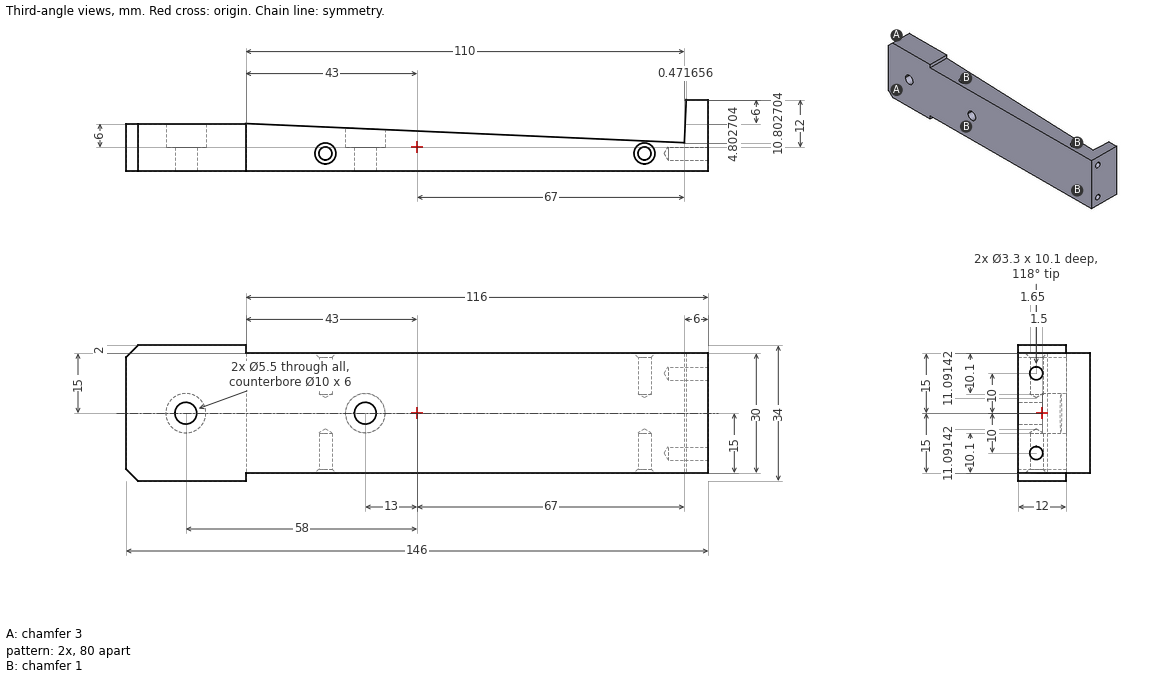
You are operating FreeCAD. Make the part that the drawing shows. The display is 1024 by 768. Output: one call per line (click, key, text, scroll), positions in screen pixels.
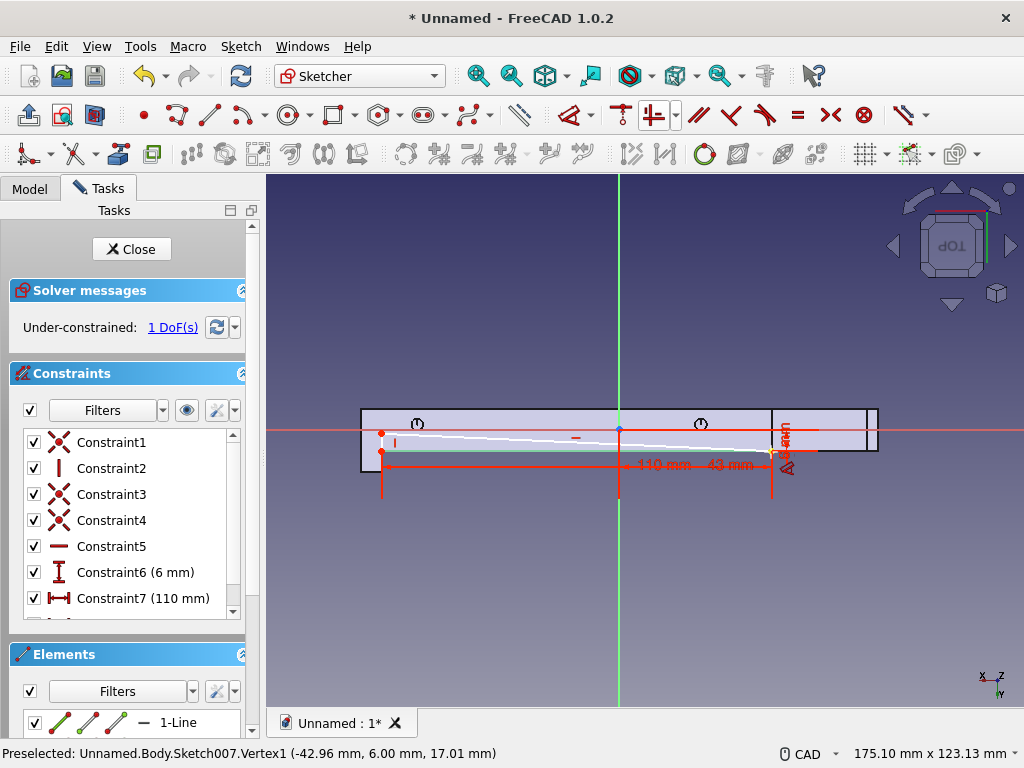
scroll(382, 439, up, 5)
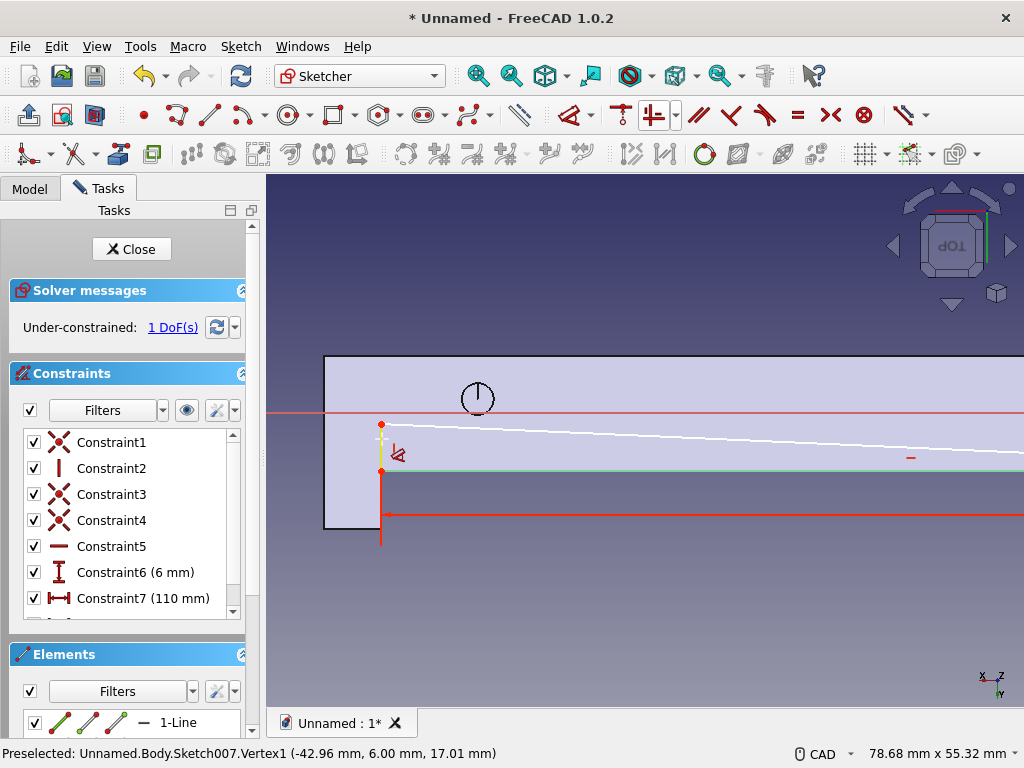
click(381, 438)
click(347, 448)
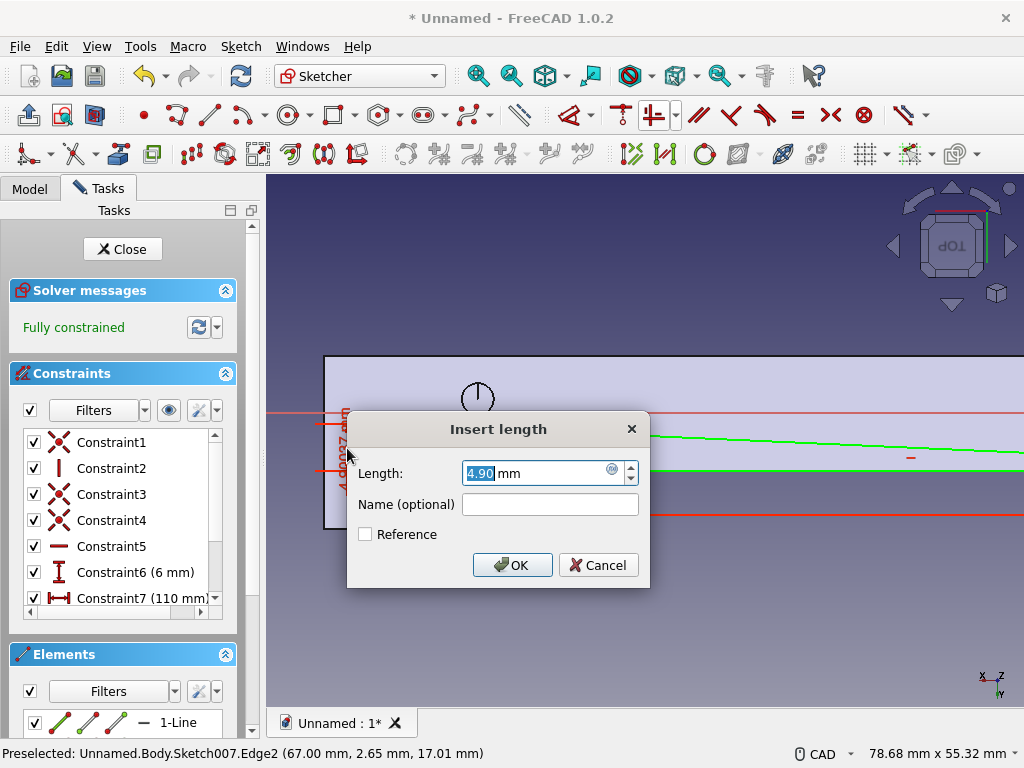
text(4.802704)
key(Return)
key(Escape)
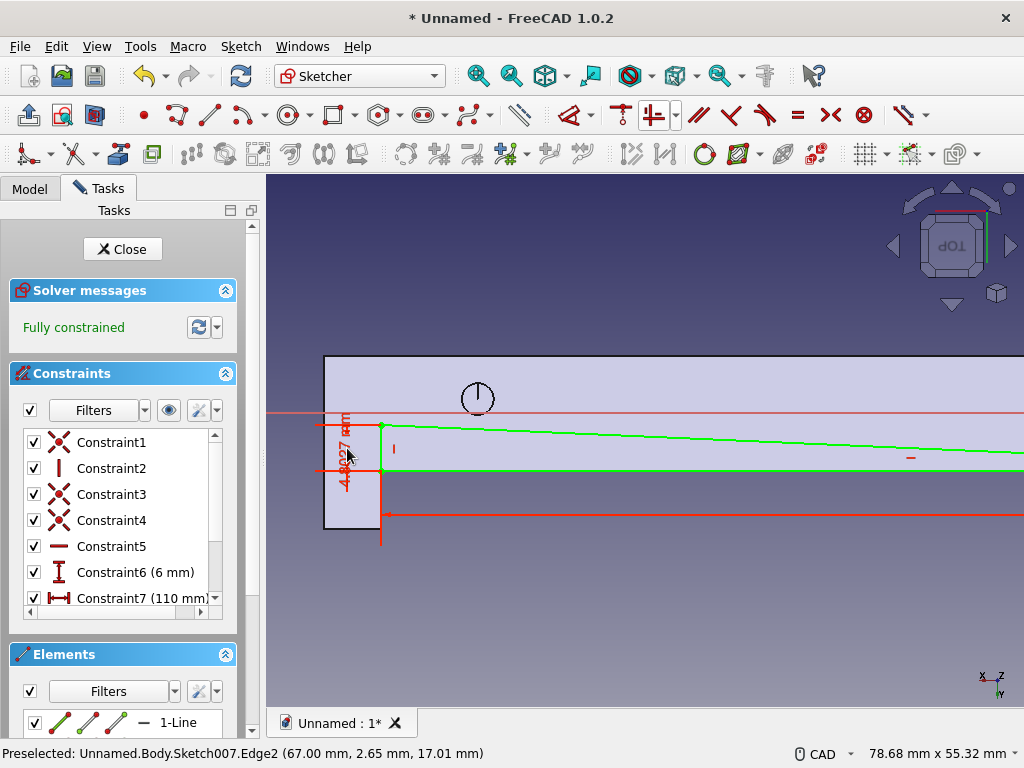
click(123, 249)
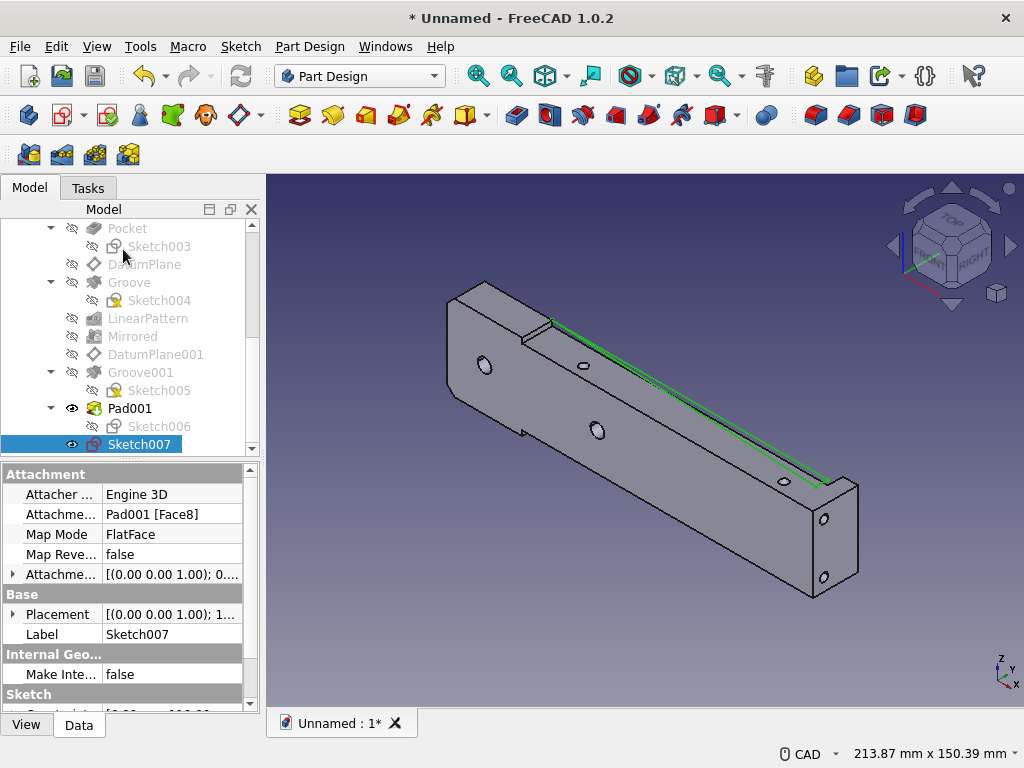
click(517, 116)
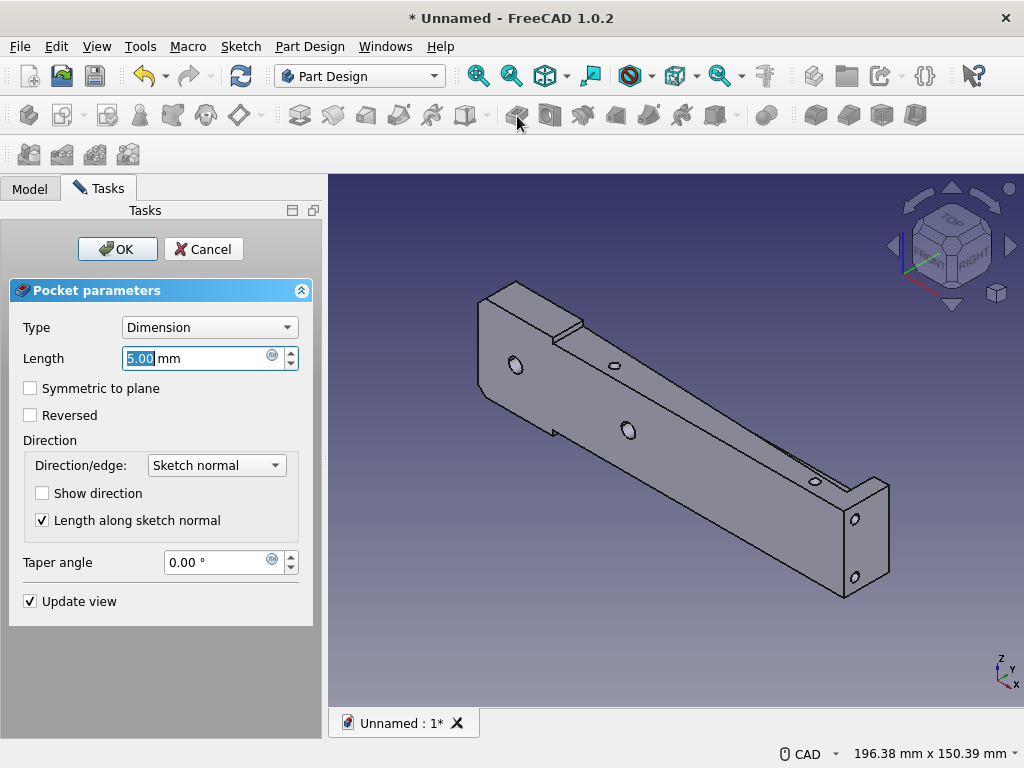
click(210, 328)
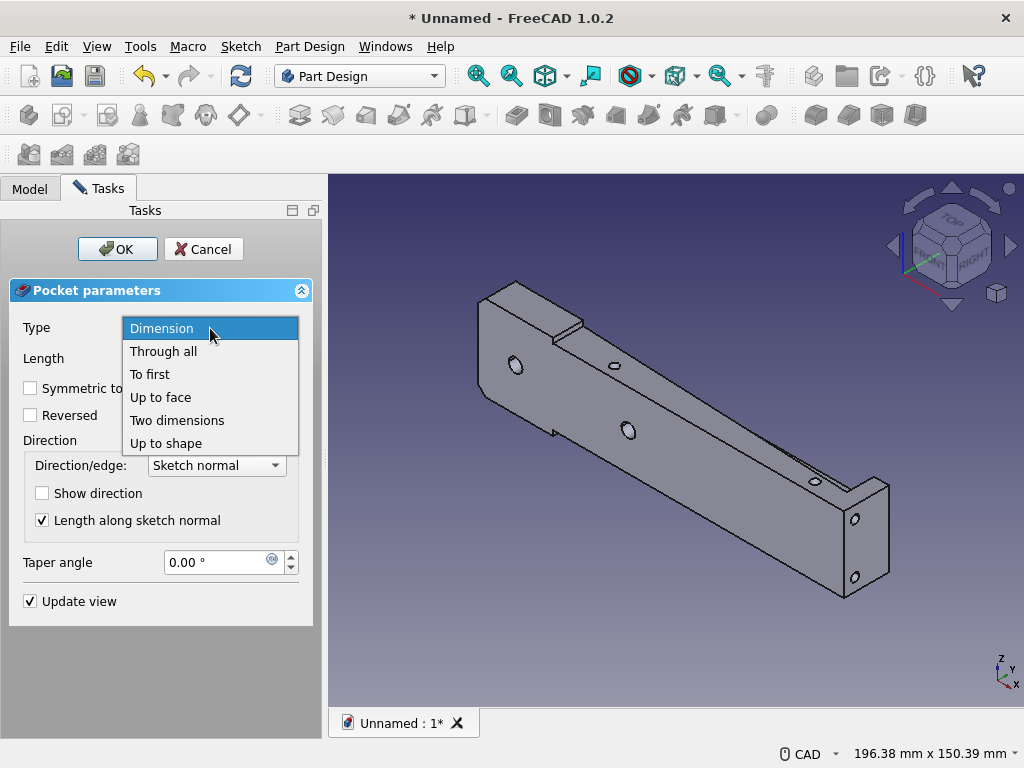
click(208, 352)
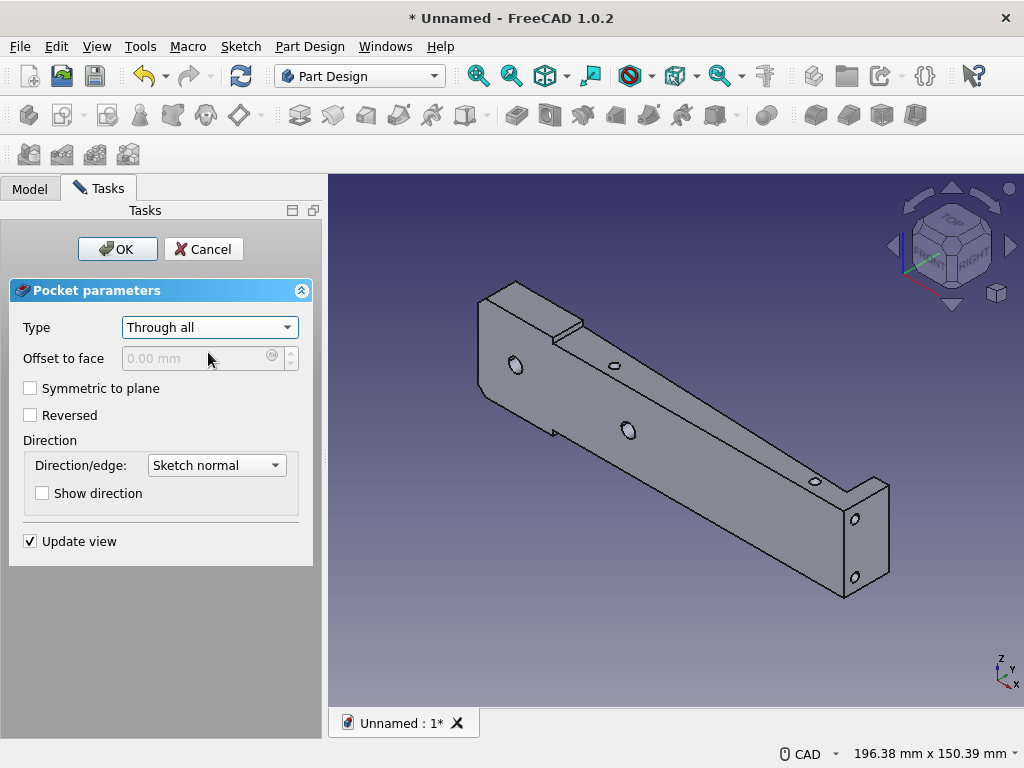
click(118, 249)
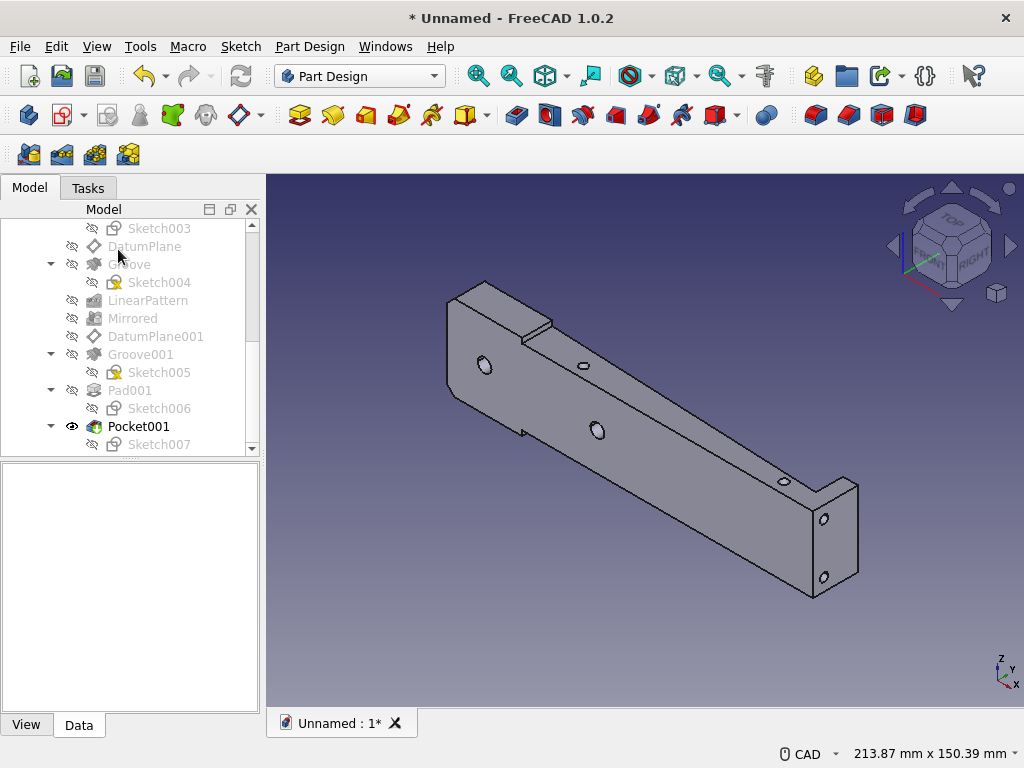
click(513, 314)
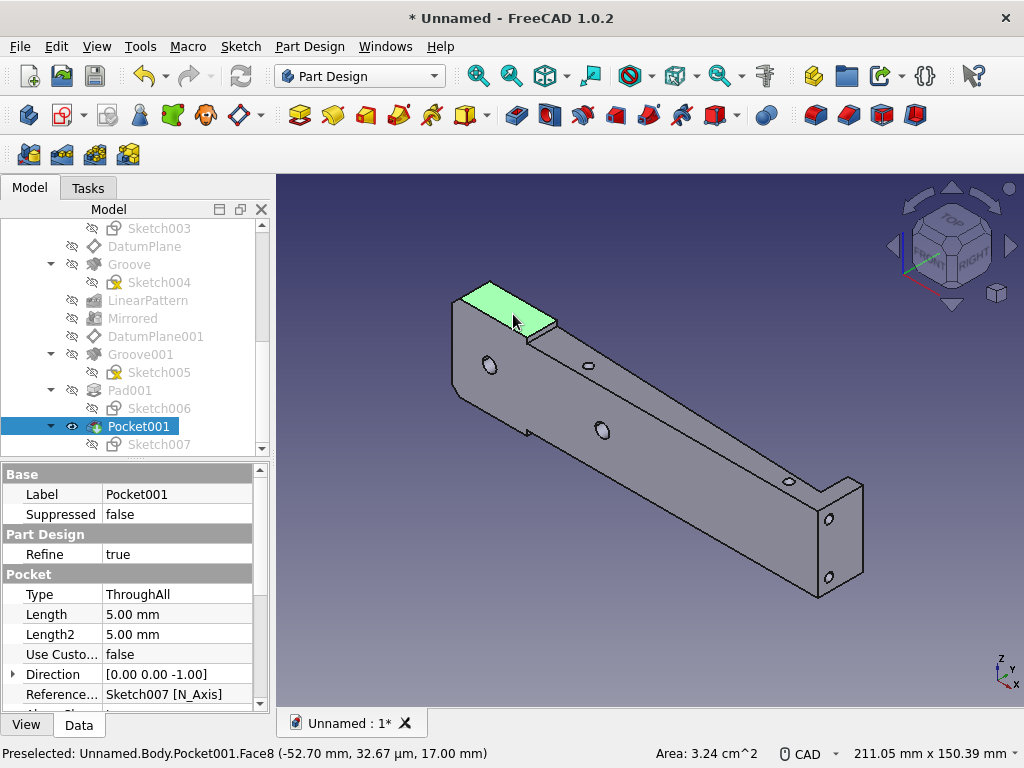
click(62, 116)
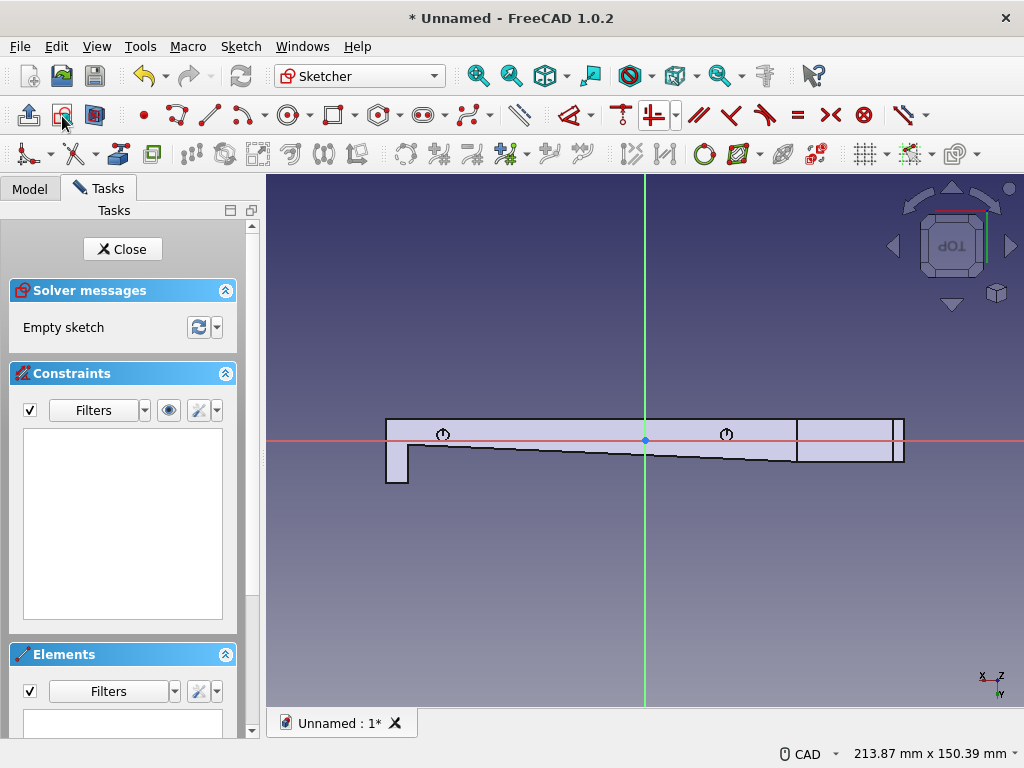
scroll(386, 467, up, 11)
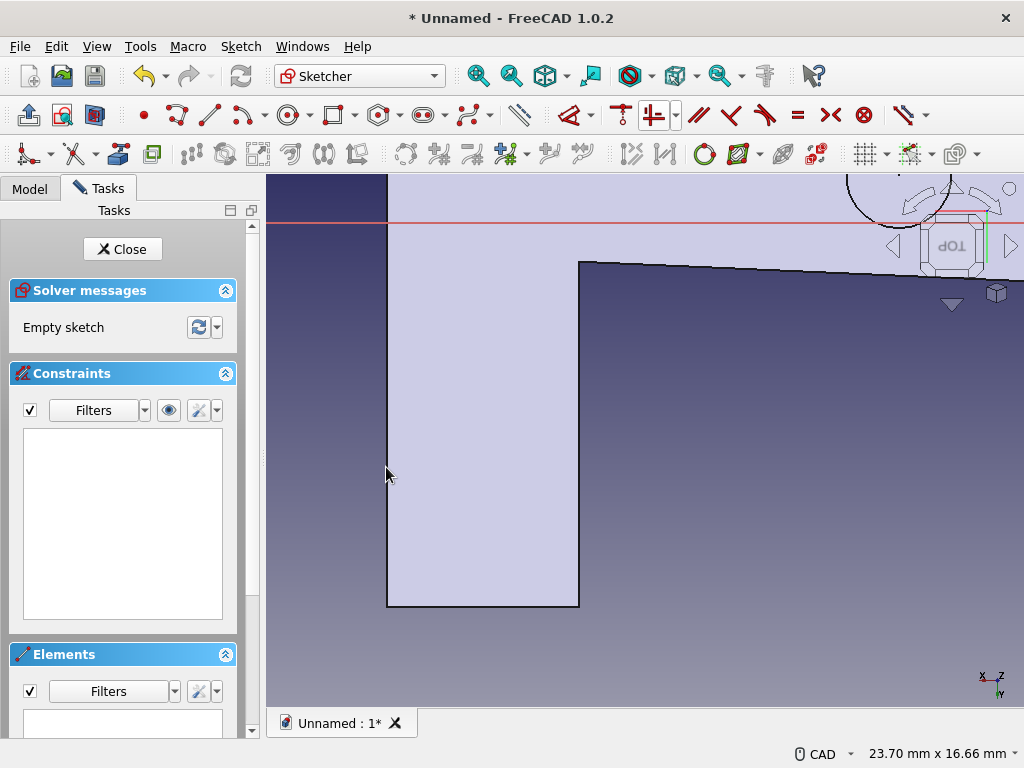
key(g)
key(m)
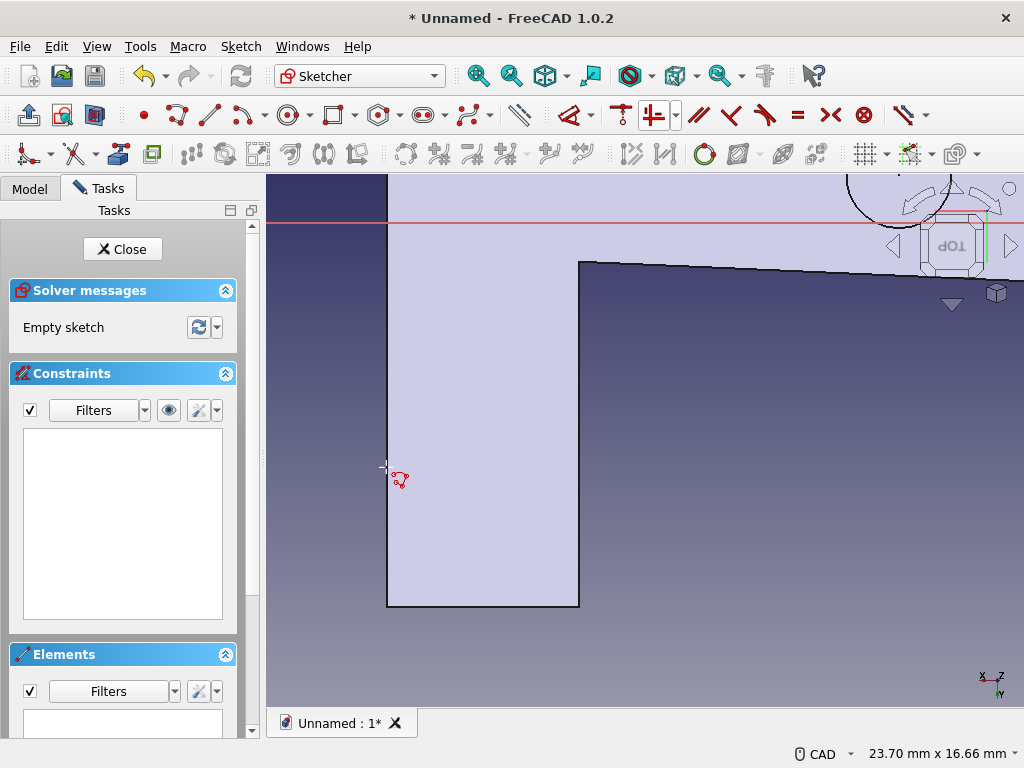
click(579, 262)
click(562, 607)
click(579, 607)
click(579, 263)
key(Escape)
key(Escape)